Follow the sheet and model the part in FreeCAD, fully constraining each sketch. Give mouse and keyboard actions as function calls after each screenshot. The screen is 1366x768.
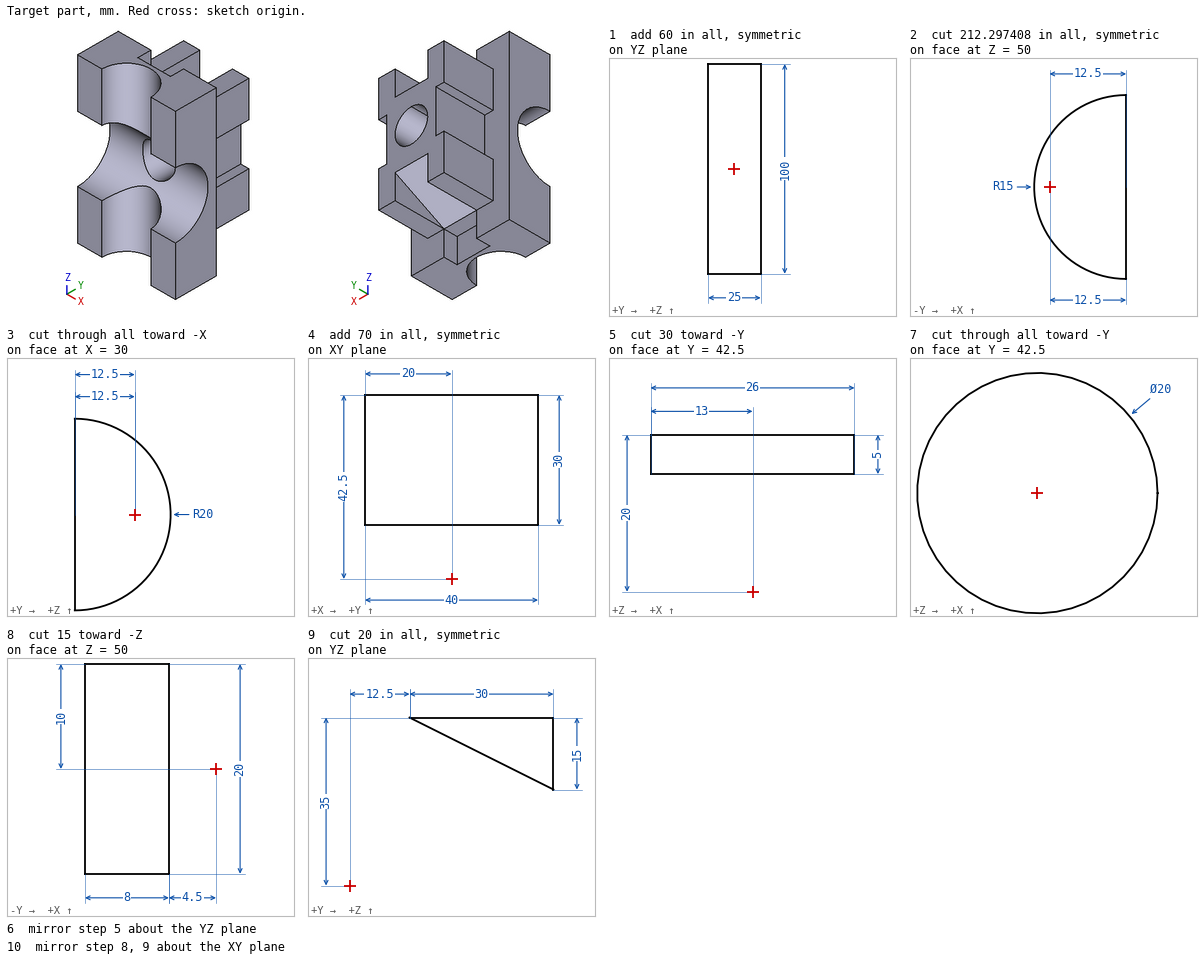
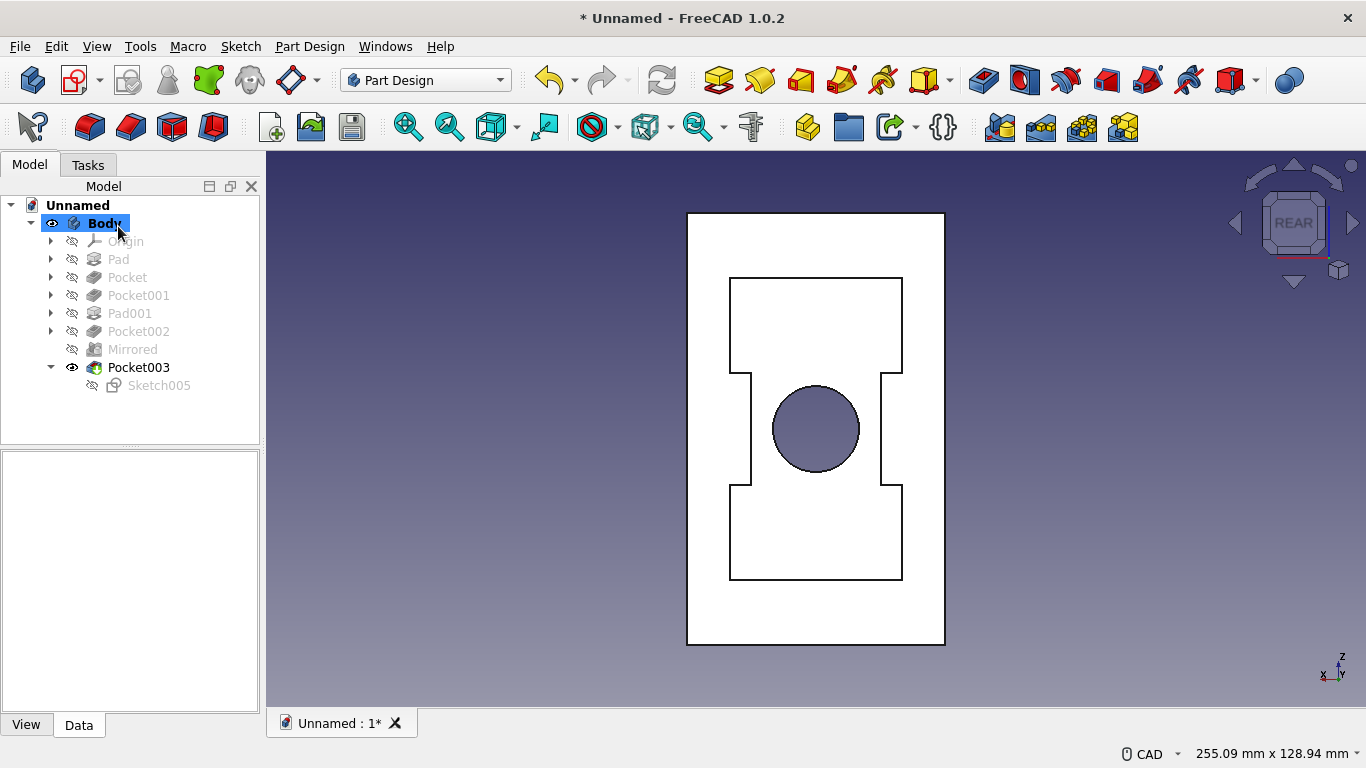
key(0)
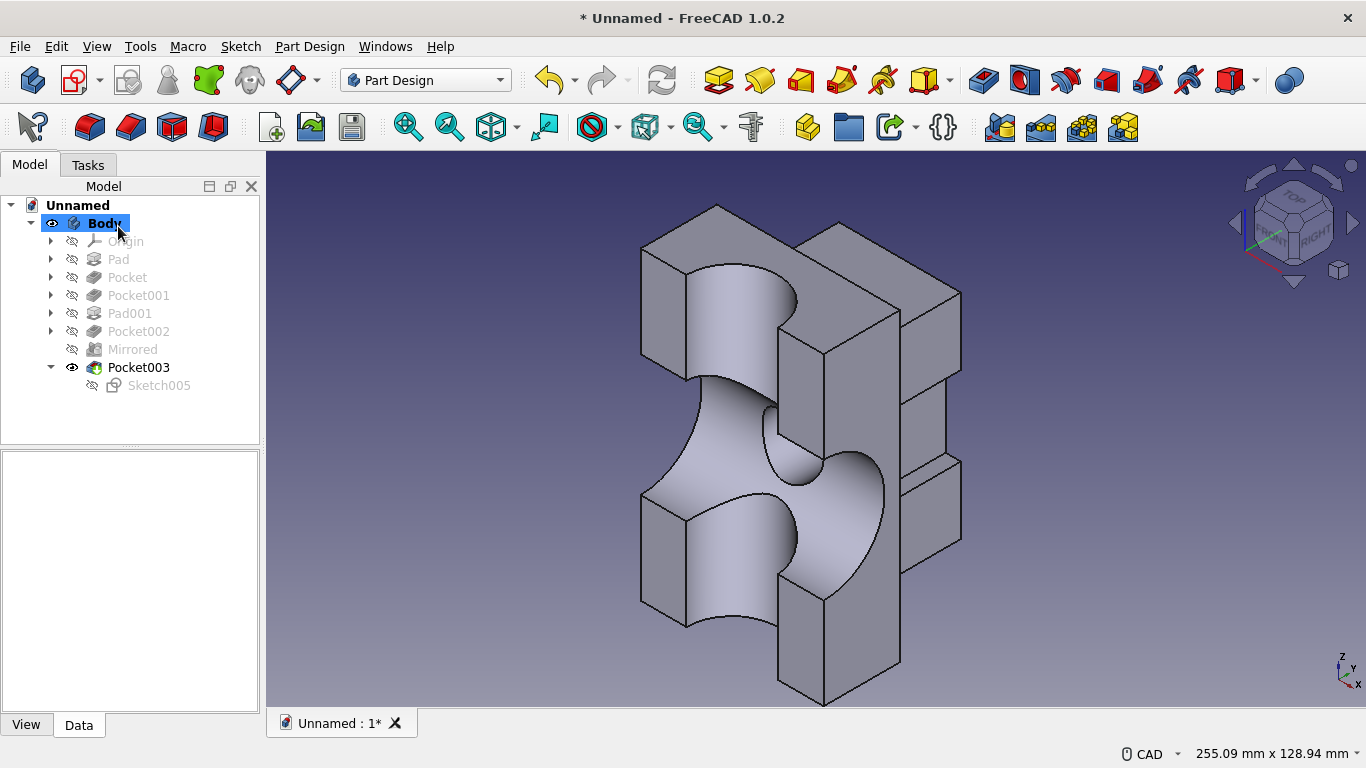
click(729, 242)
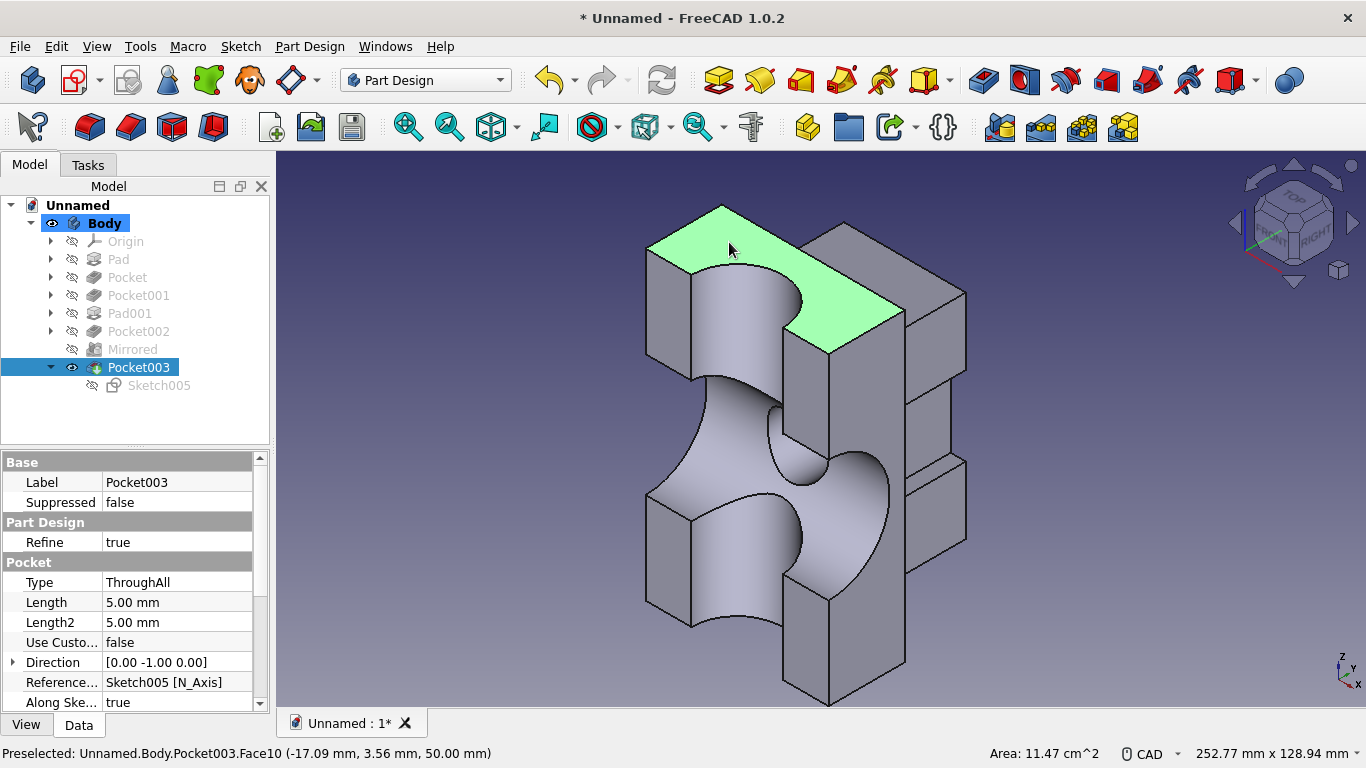
click(74, 80)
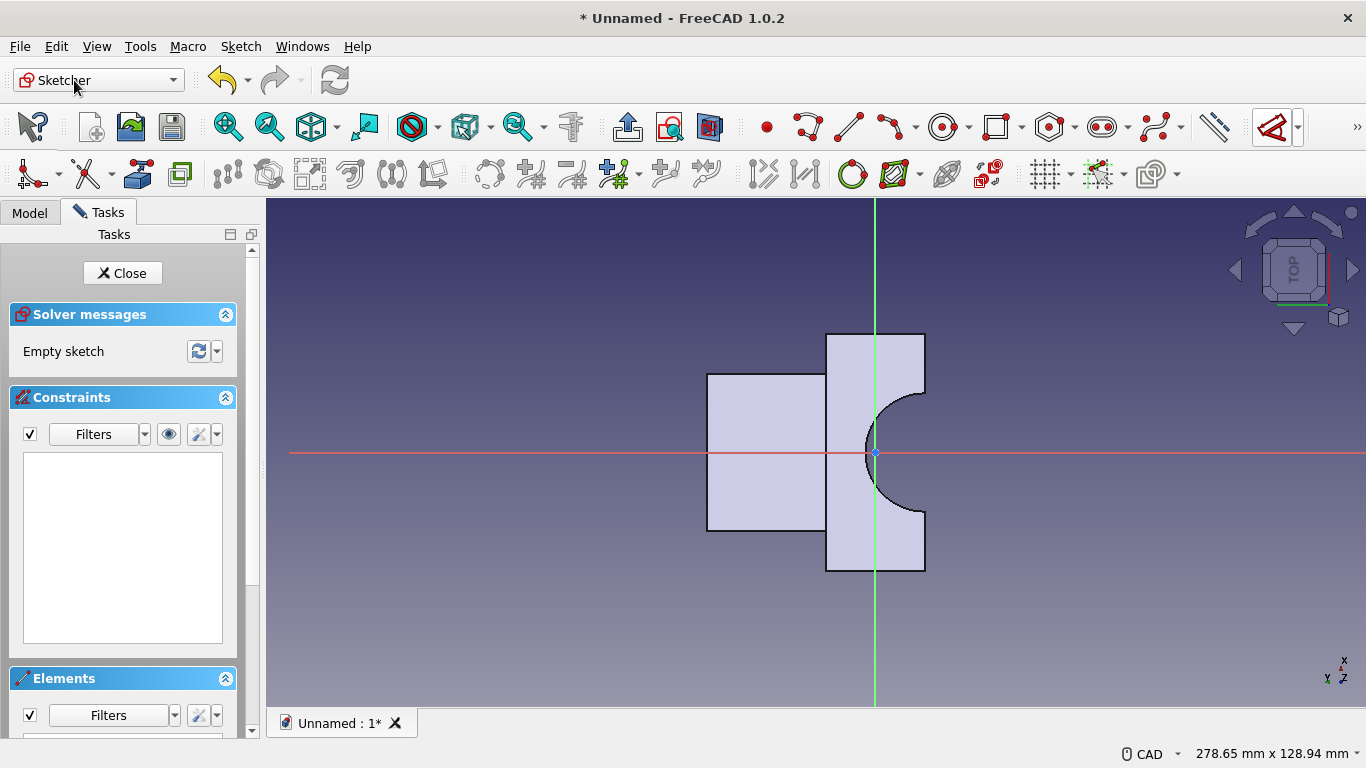
scroll(884, 453, up, 7)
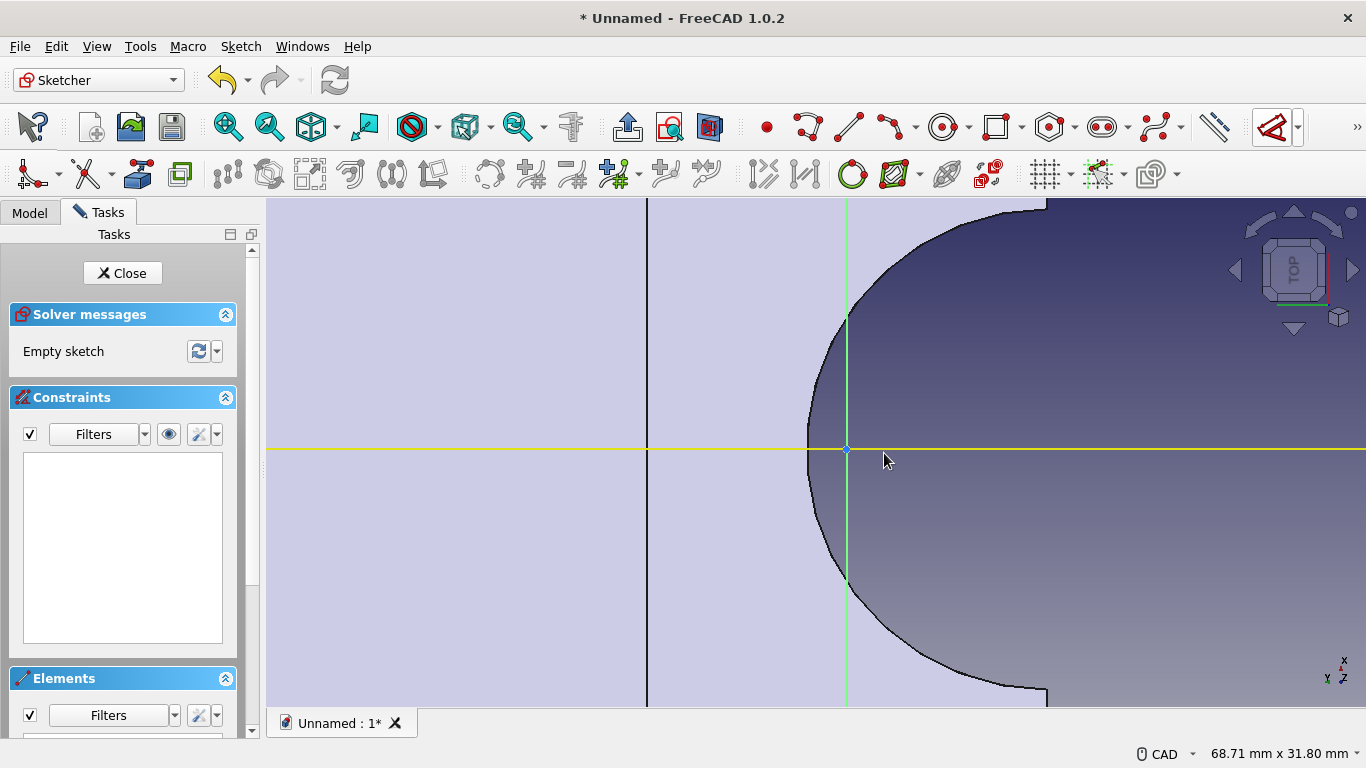
key(g)
key(r)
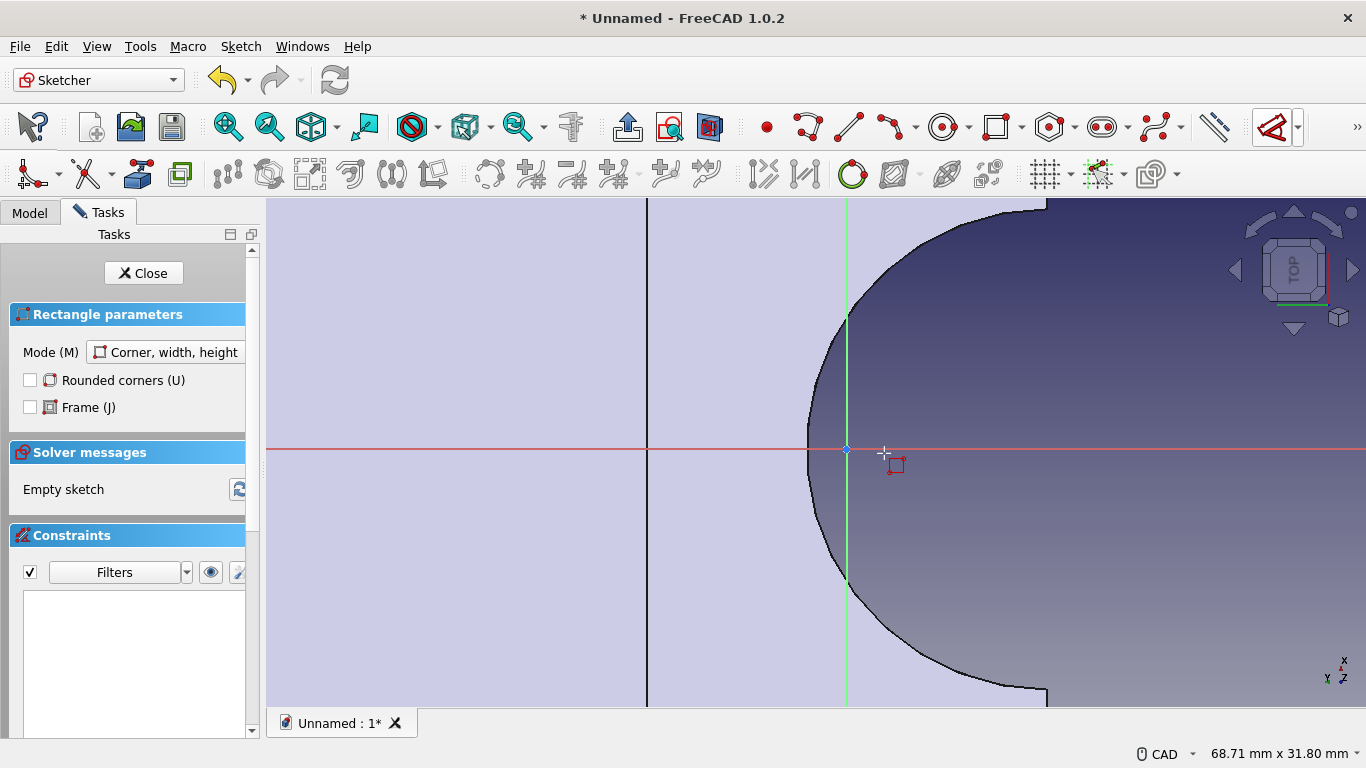
click(647, 289)
move(775, 610)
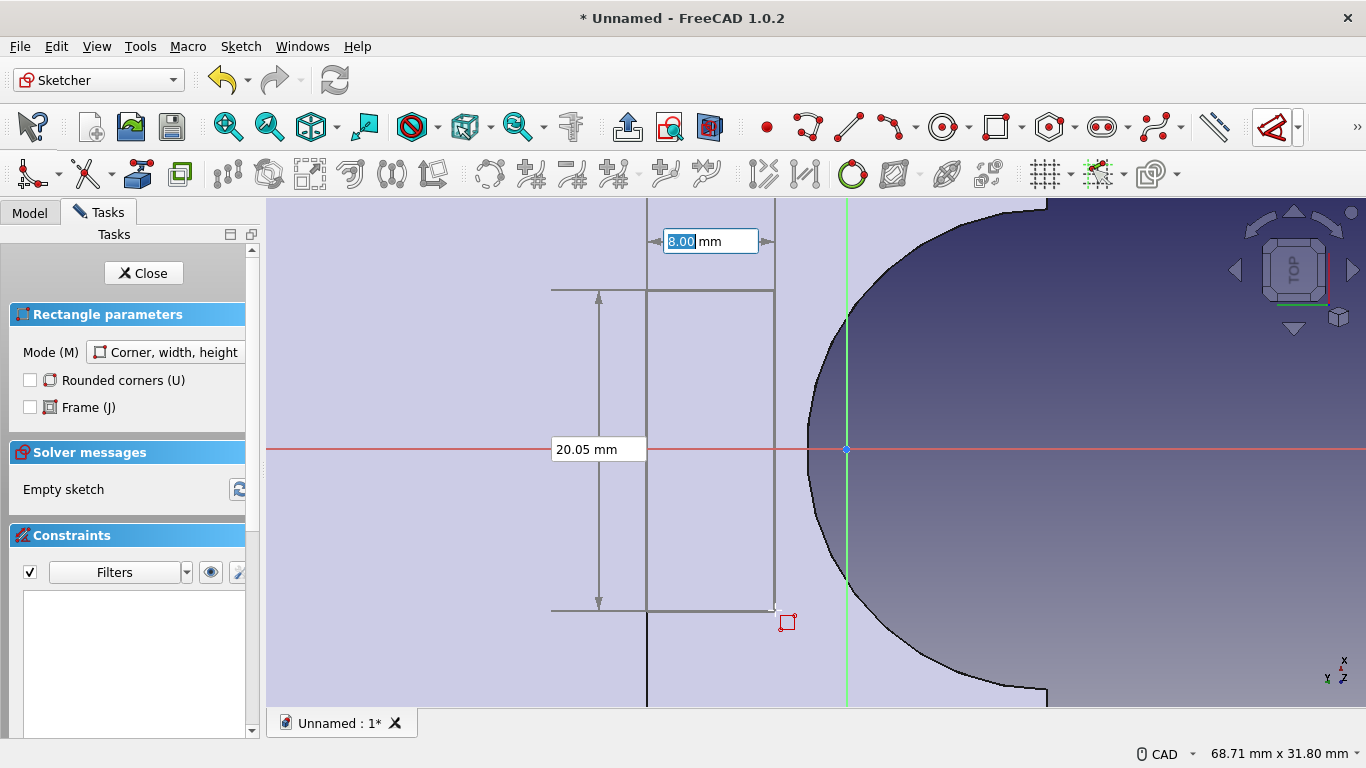
text(8)
key(Tab)
text(20)
key(Return)
key(Escape)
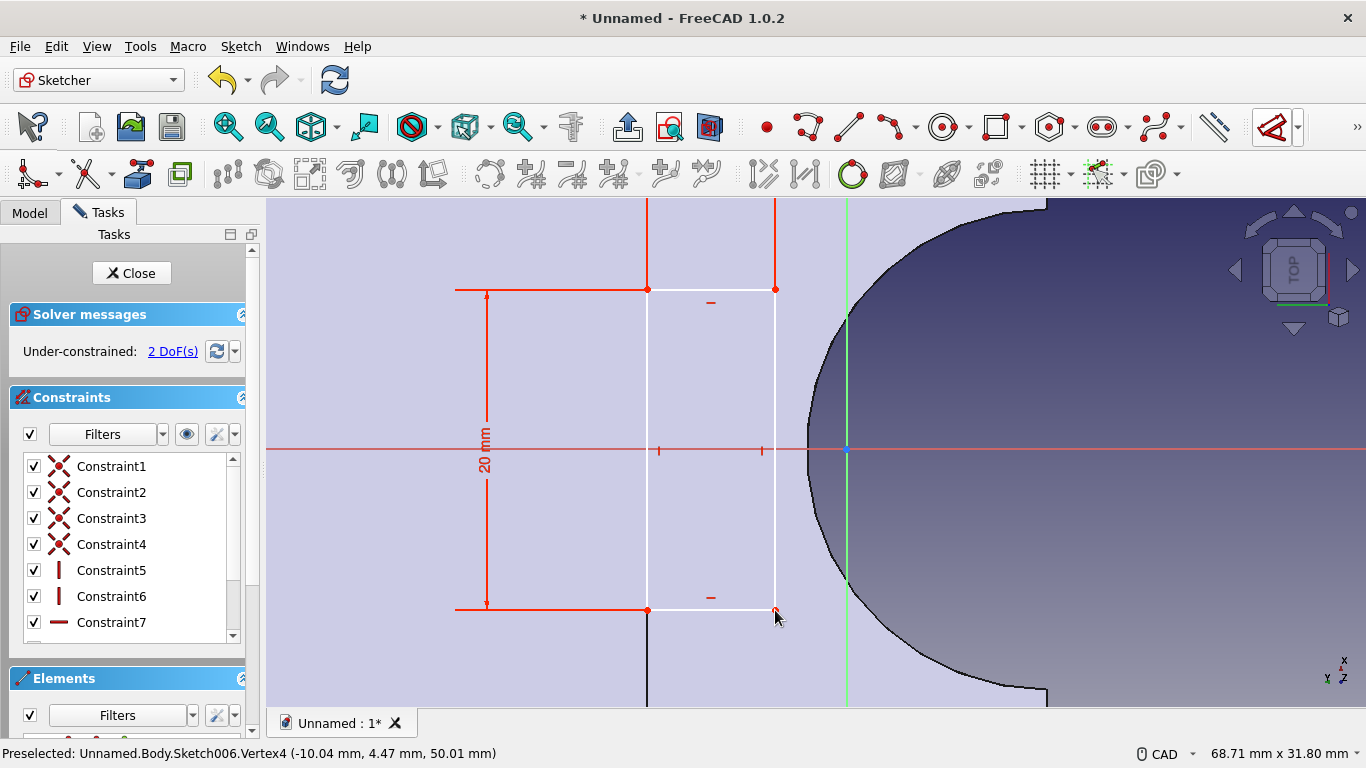
click(647, 290)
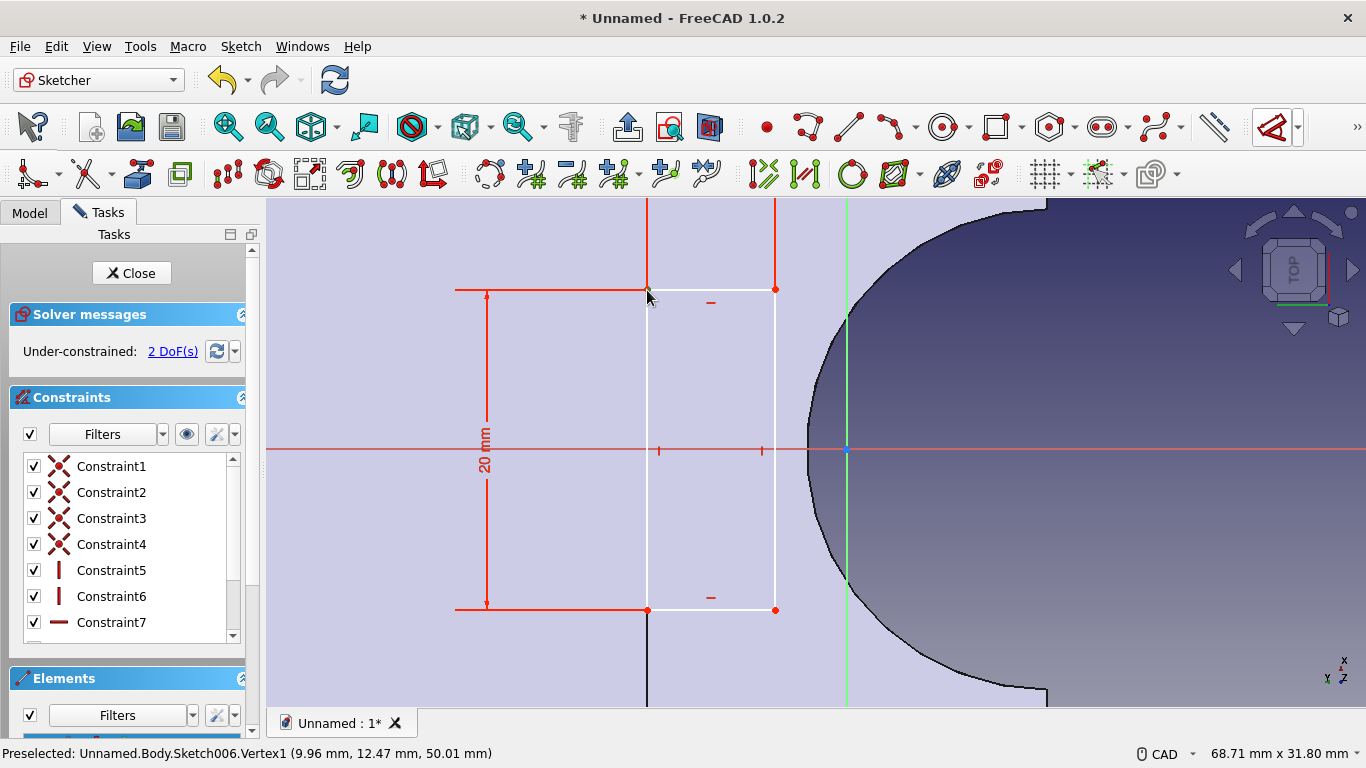
key(i)